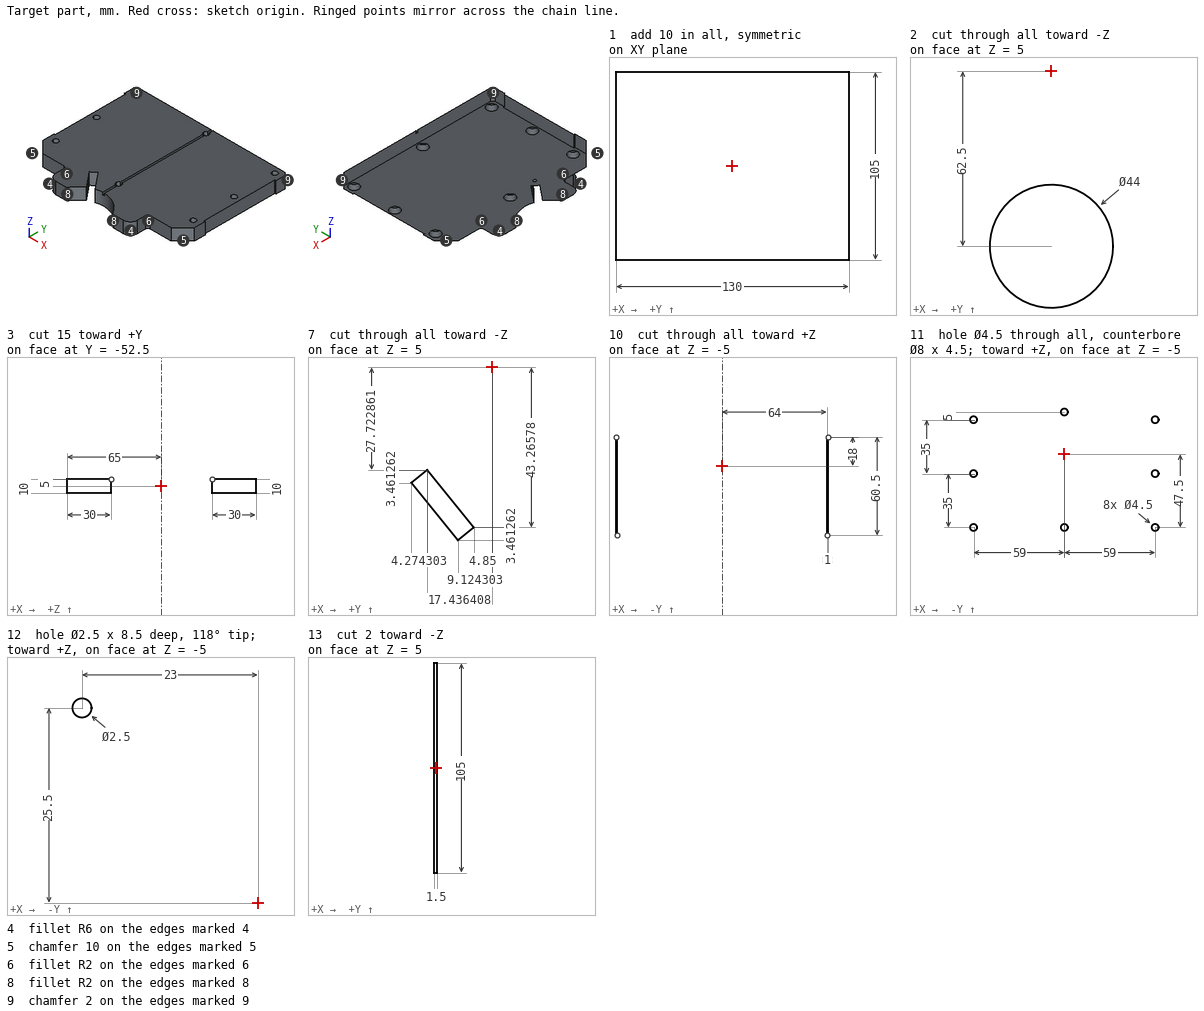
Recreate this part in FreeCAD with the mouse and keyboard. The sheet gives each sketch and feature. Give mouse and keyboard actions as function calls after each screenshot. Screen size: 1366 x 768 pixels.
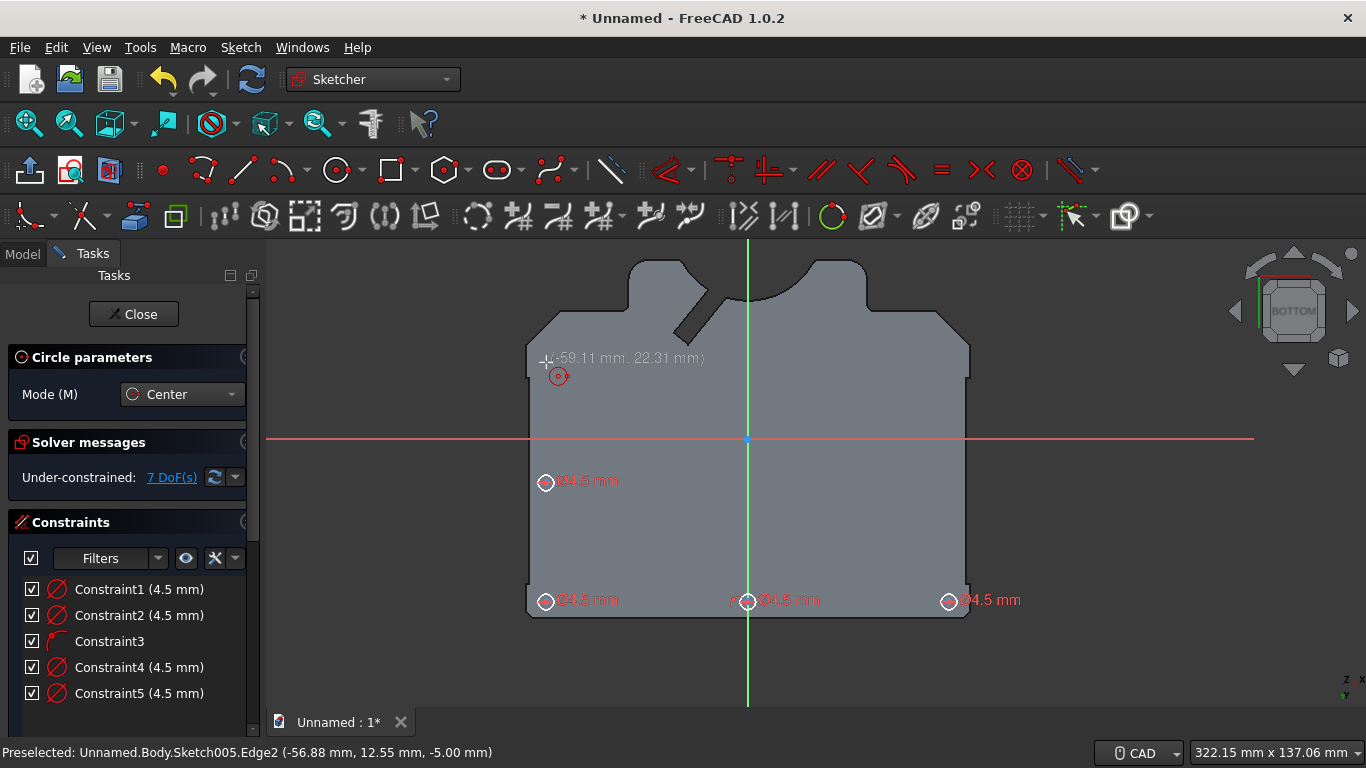
click(546, 362)
move(552, 357)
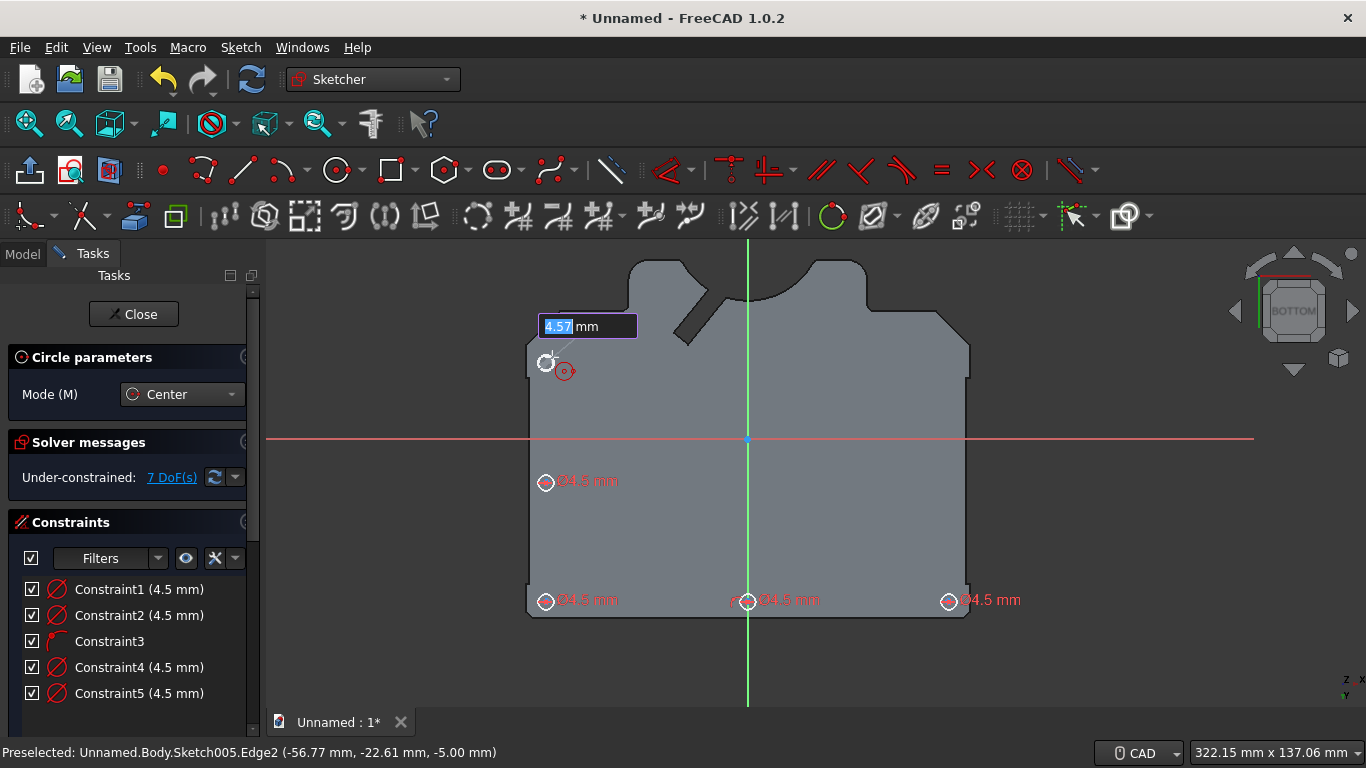
text(4.5)
key(Return)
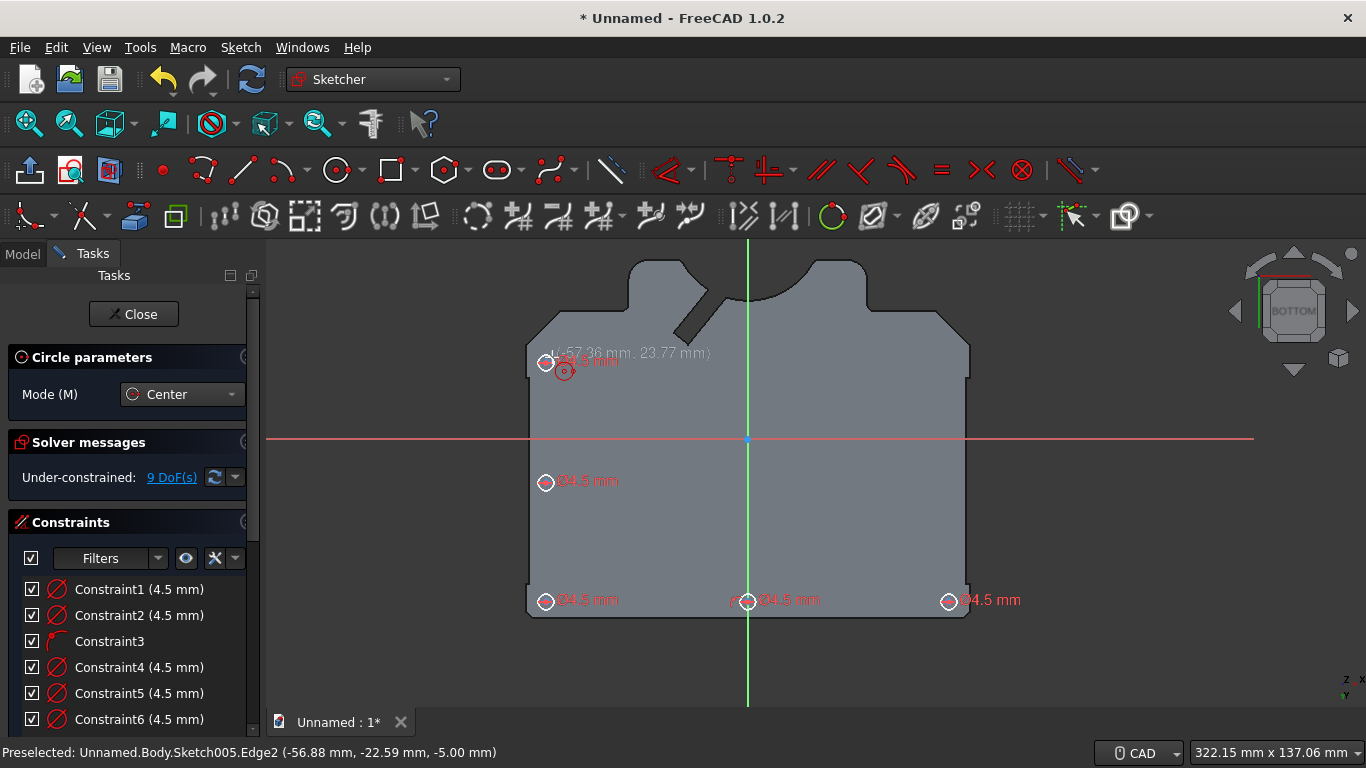
scroll(748, 345, up, 6)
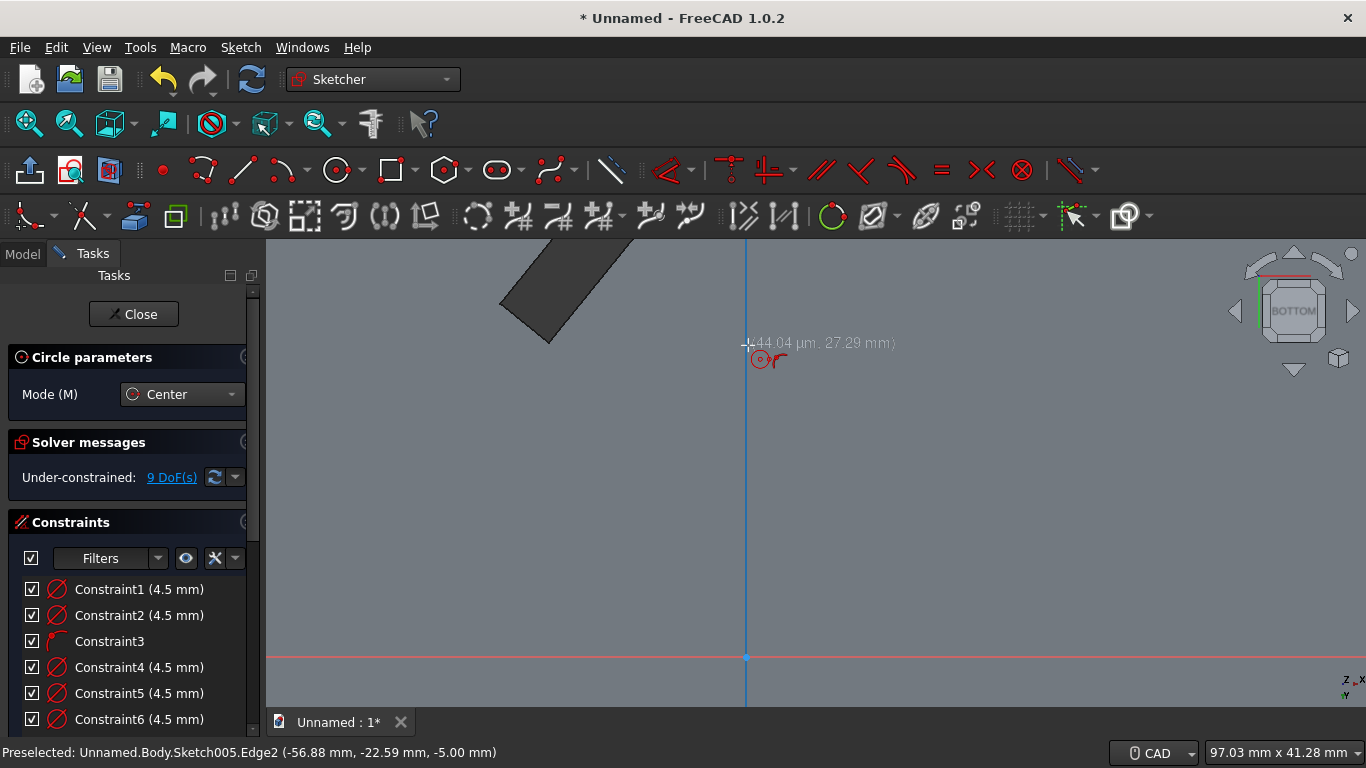
scroll(748, 345, down, 6)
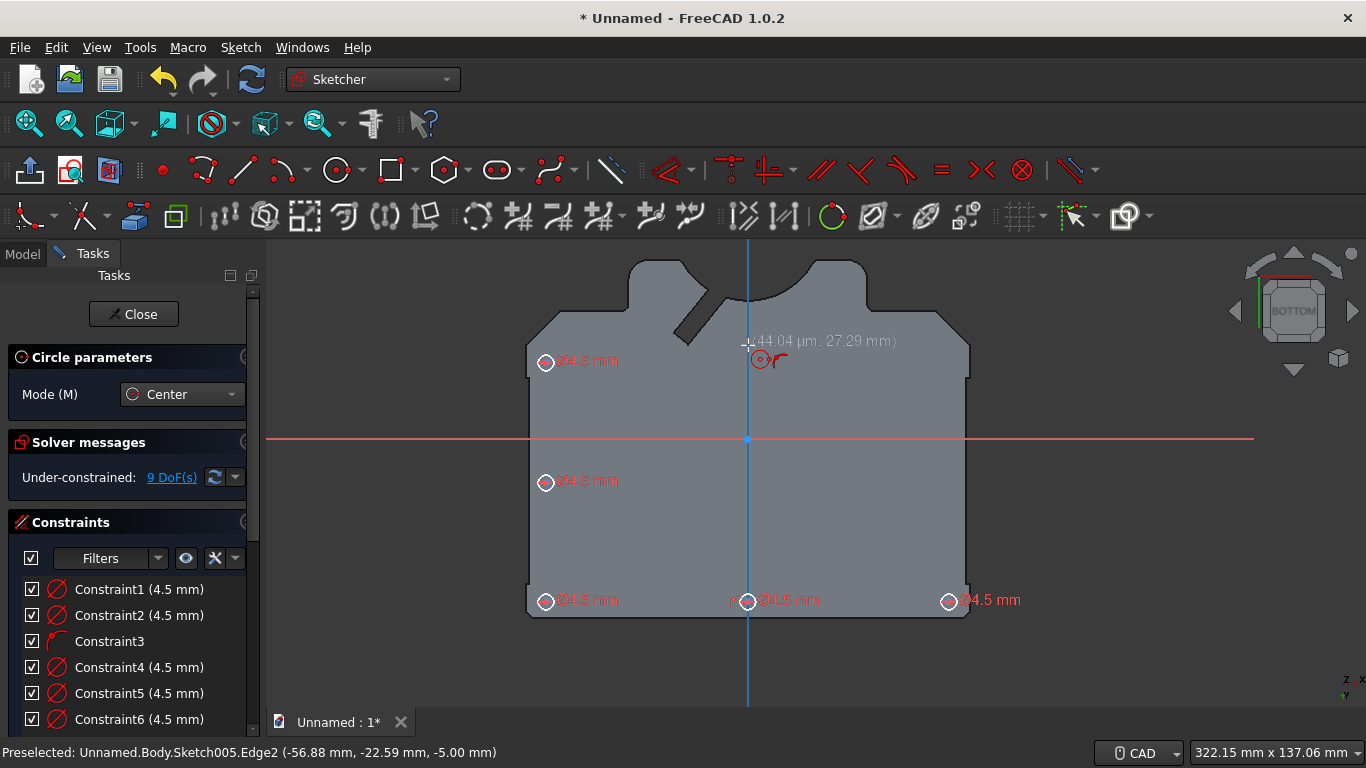
click(748, 345)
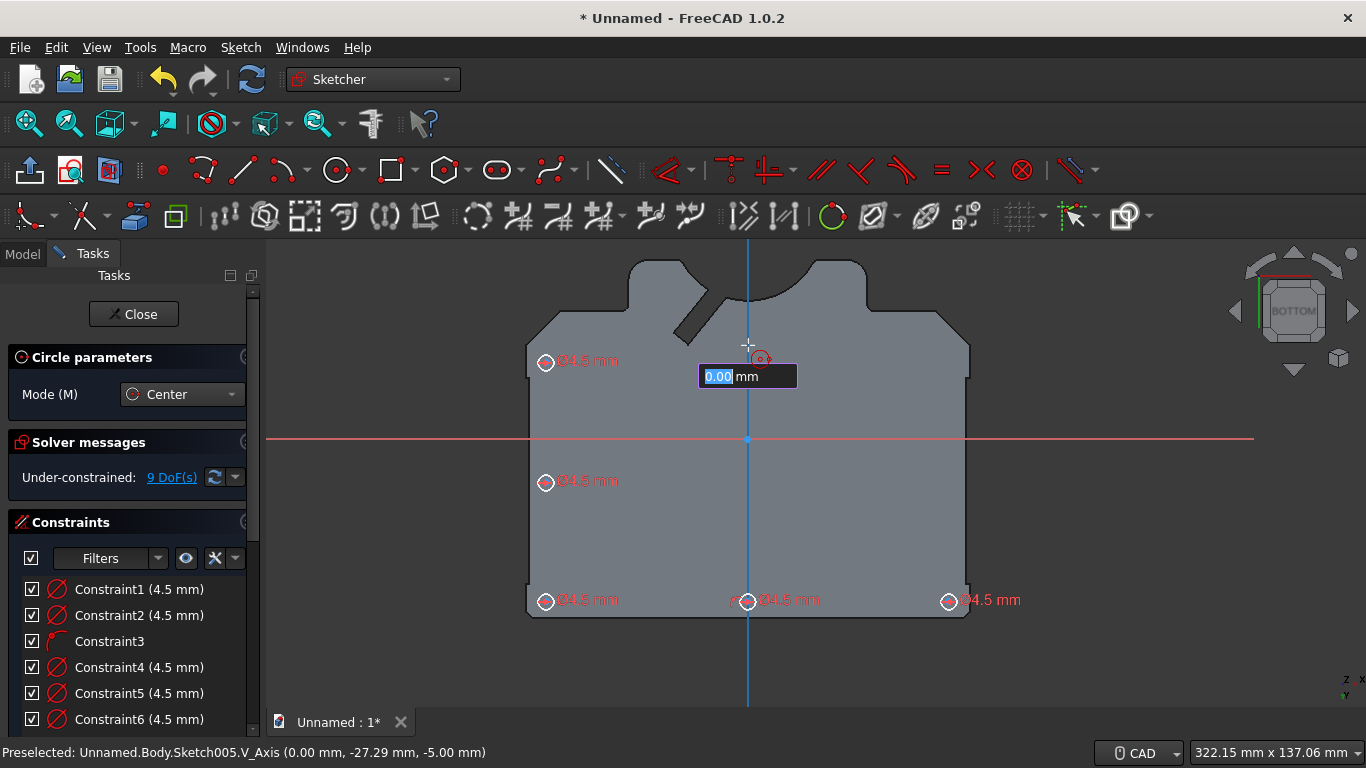
scroll(755, 343, up, 4)
move(755, 342)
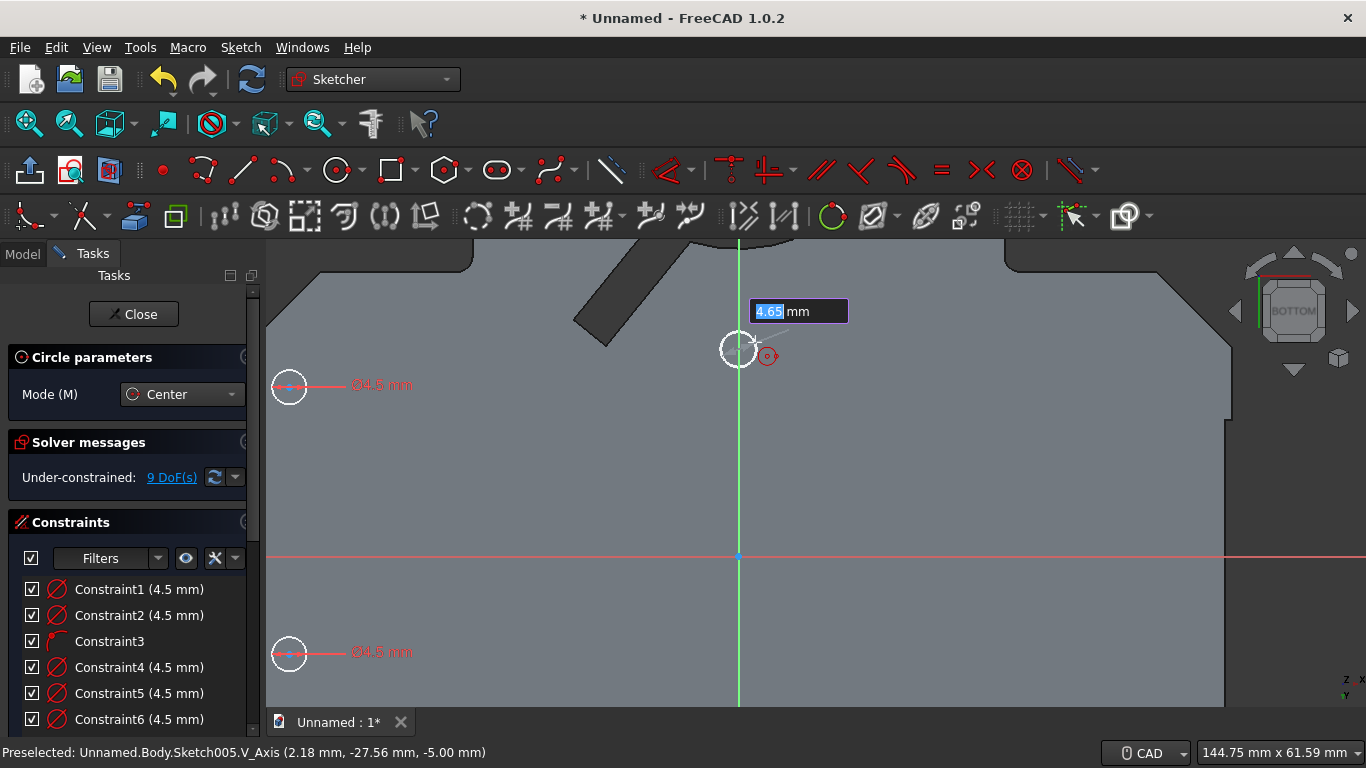
text(4.5)
key(Return)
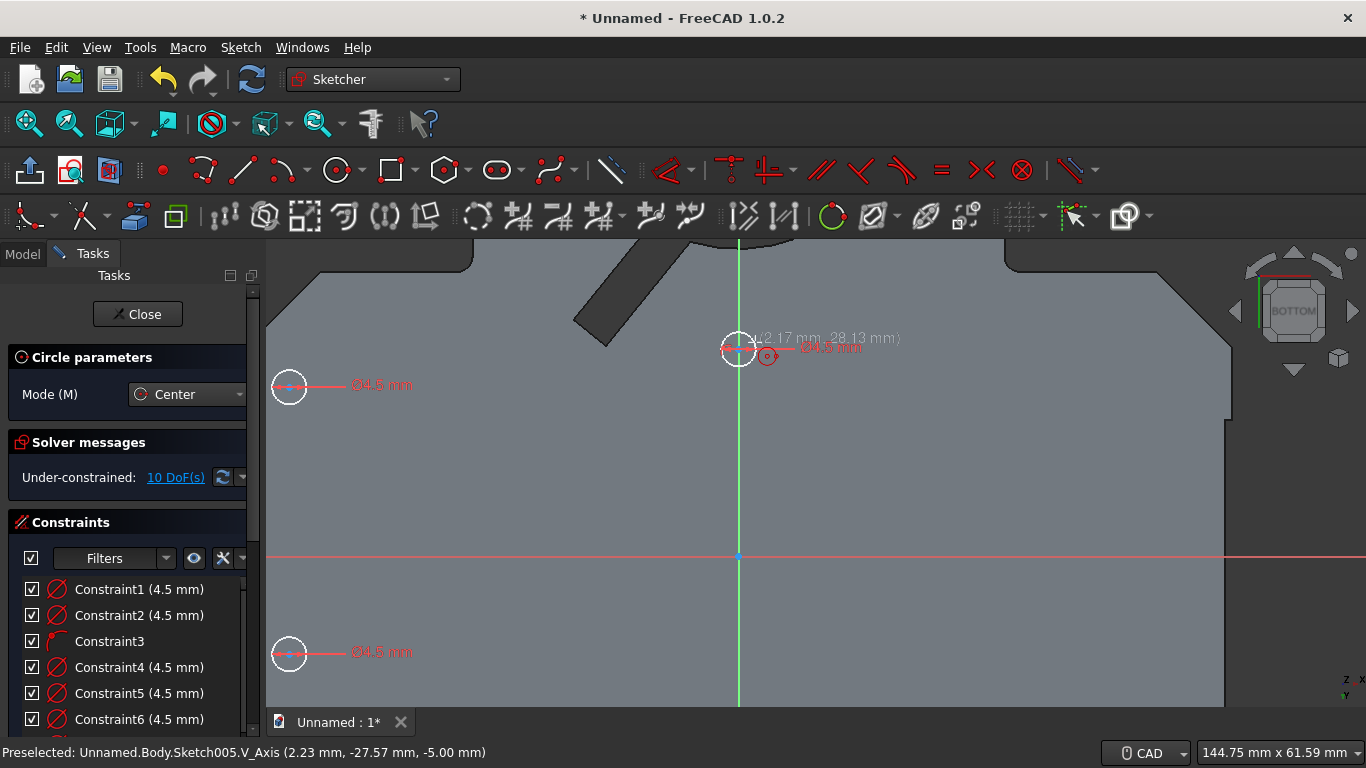
scroll(1187, 386, up, 2)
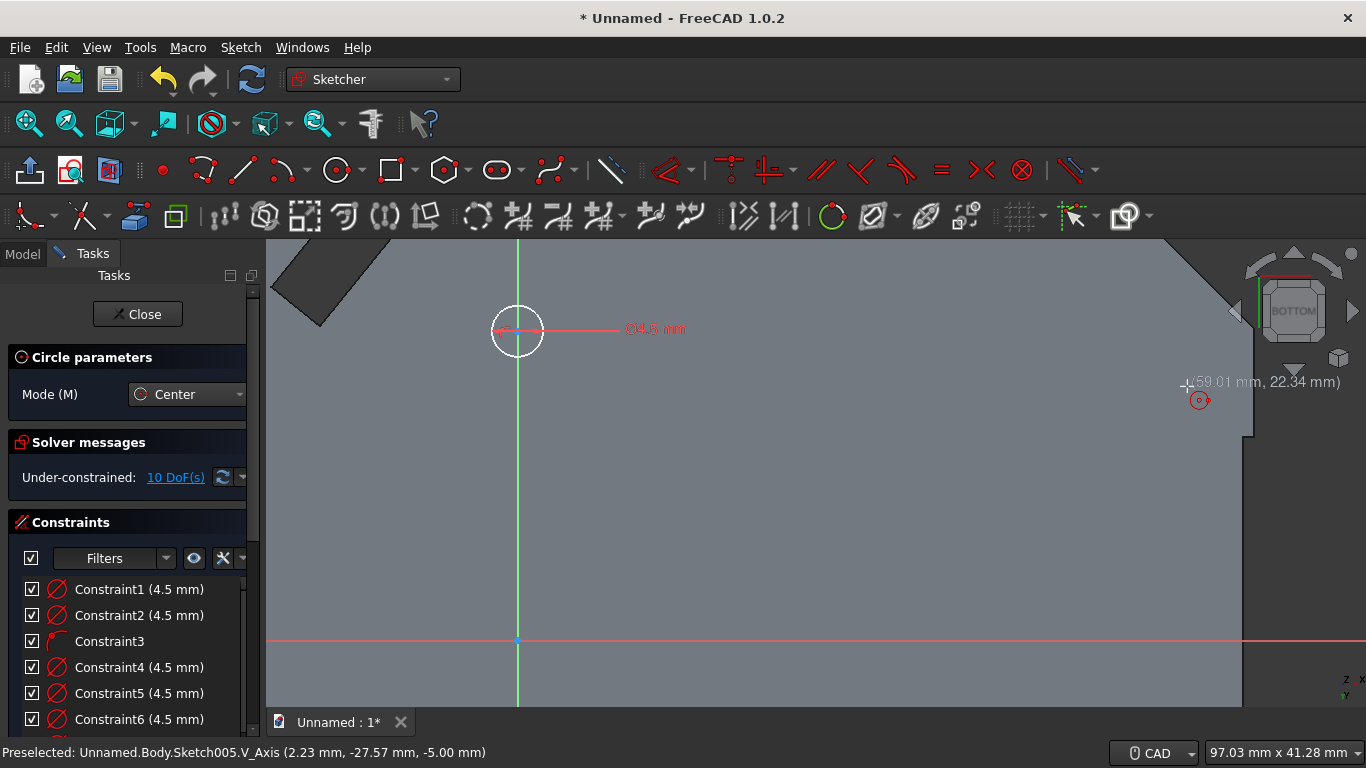
scroll(847, 352, down, 6)